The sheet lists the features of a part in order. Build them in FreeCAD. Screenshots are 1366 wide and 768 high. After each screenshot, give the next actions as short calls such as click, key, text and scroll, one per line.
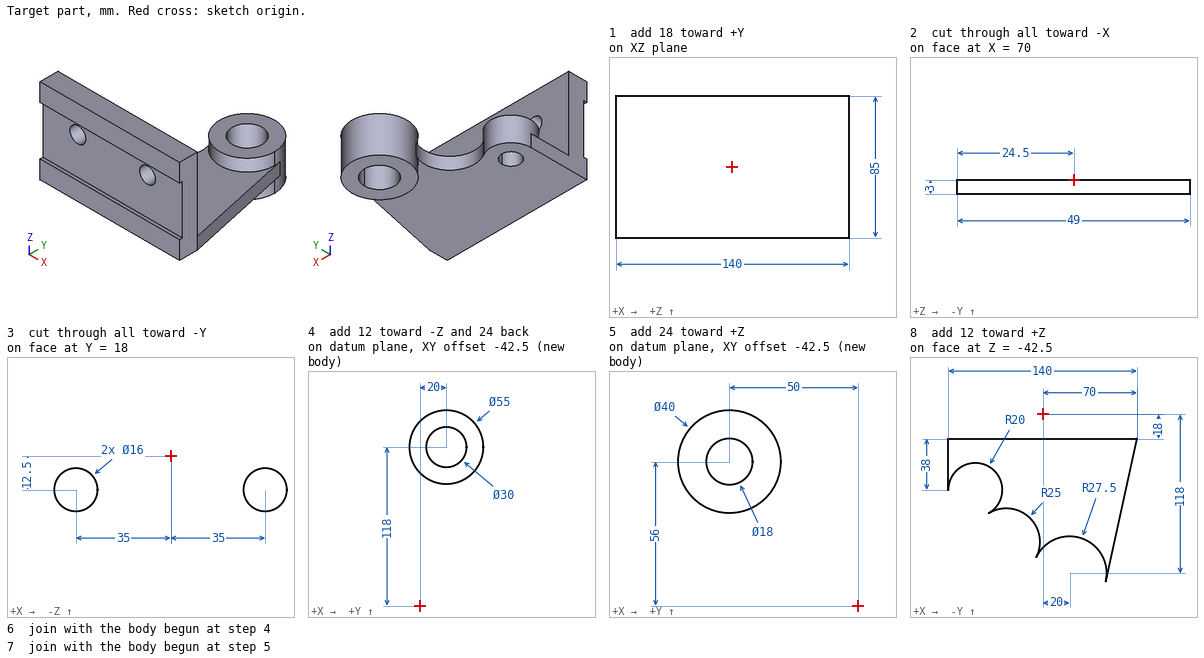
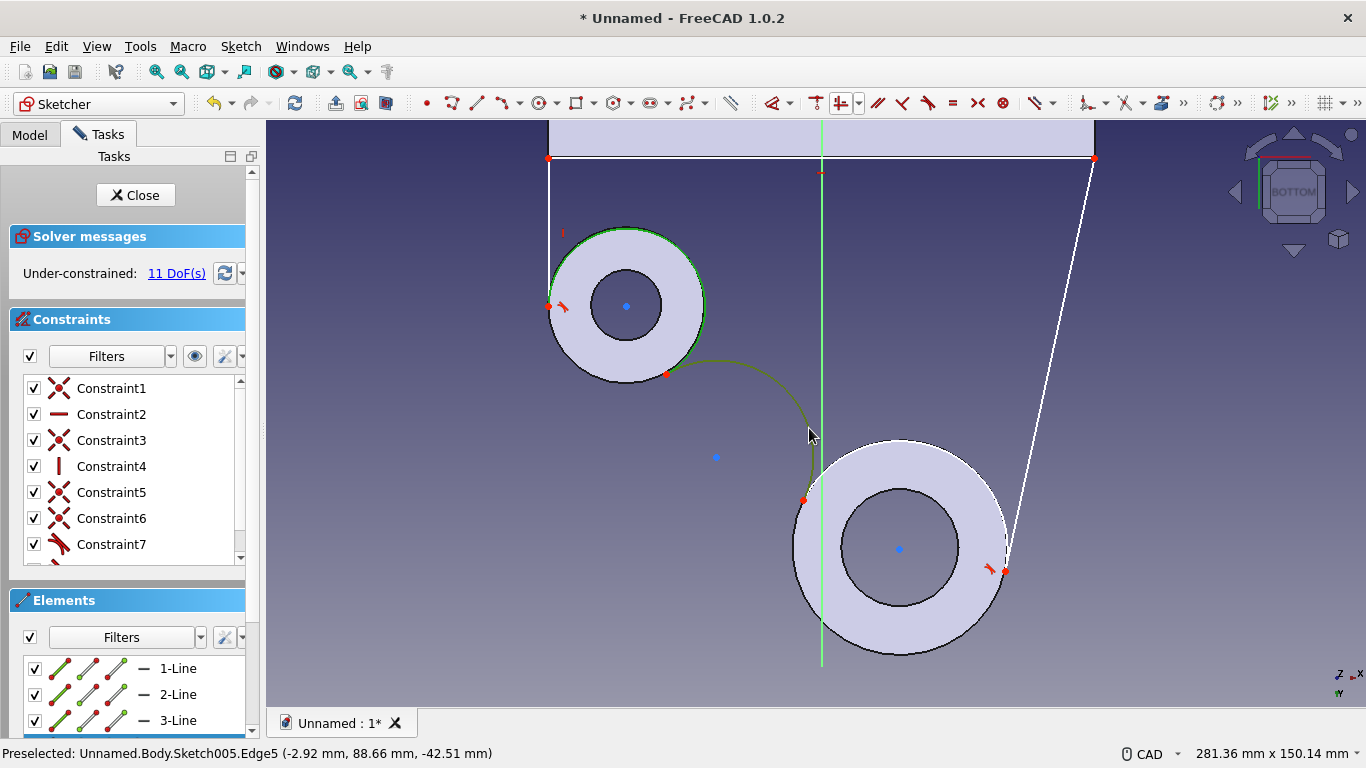
click(928, 104)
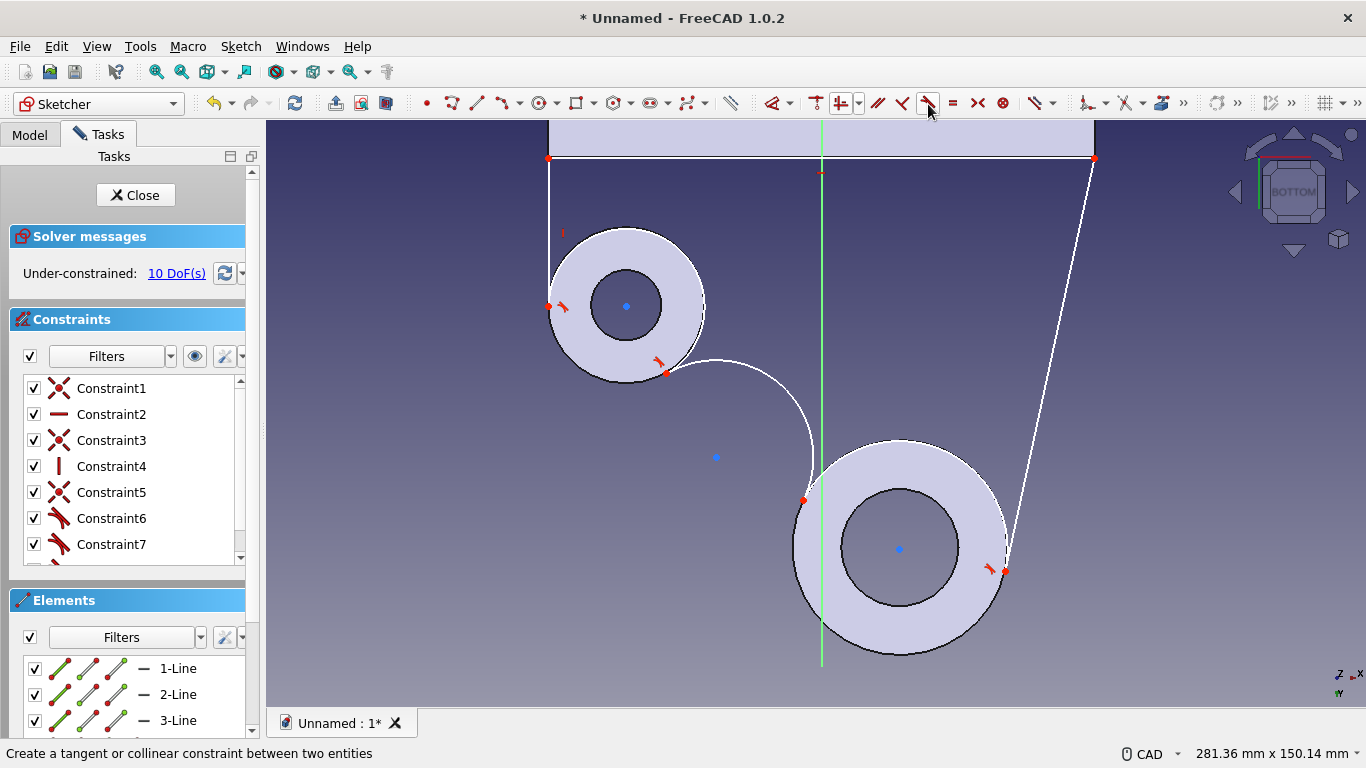
click(809, 428)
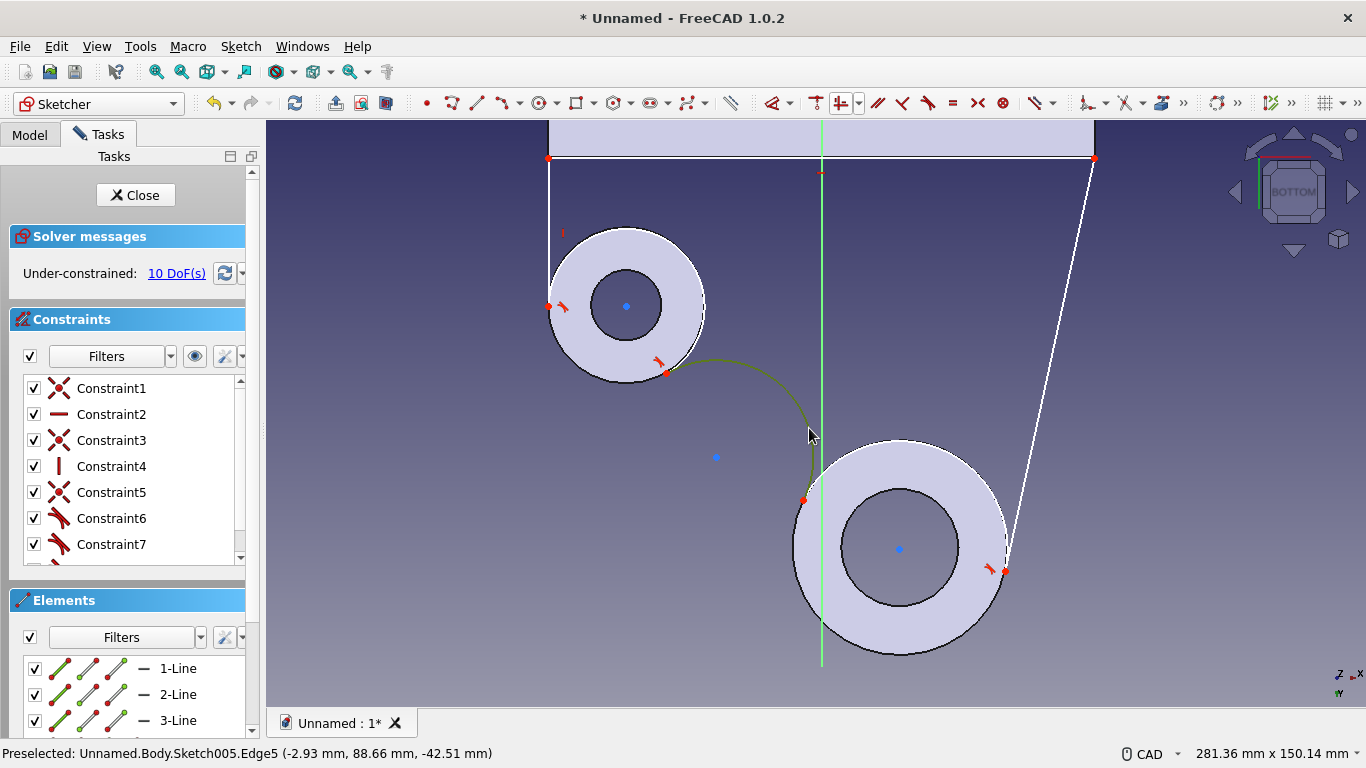
click(985, 483)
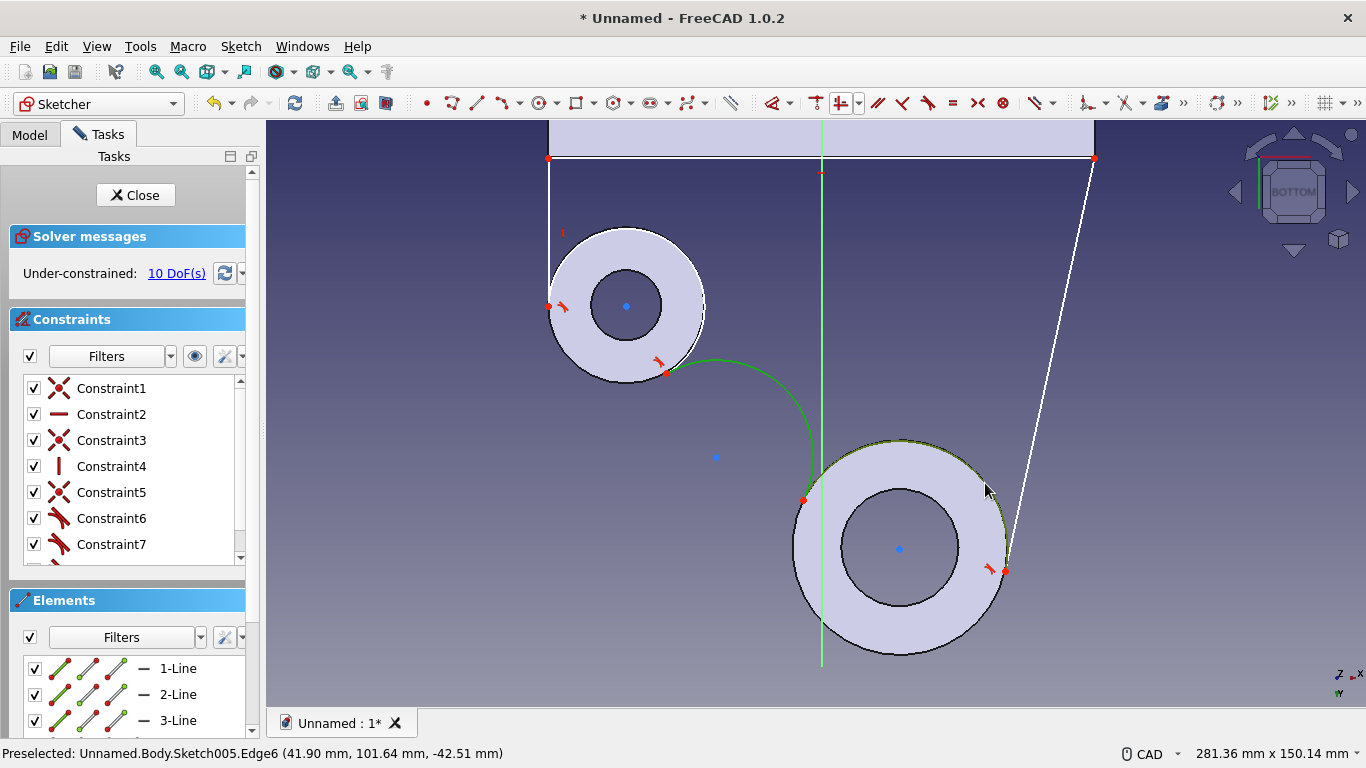
click(928, 104)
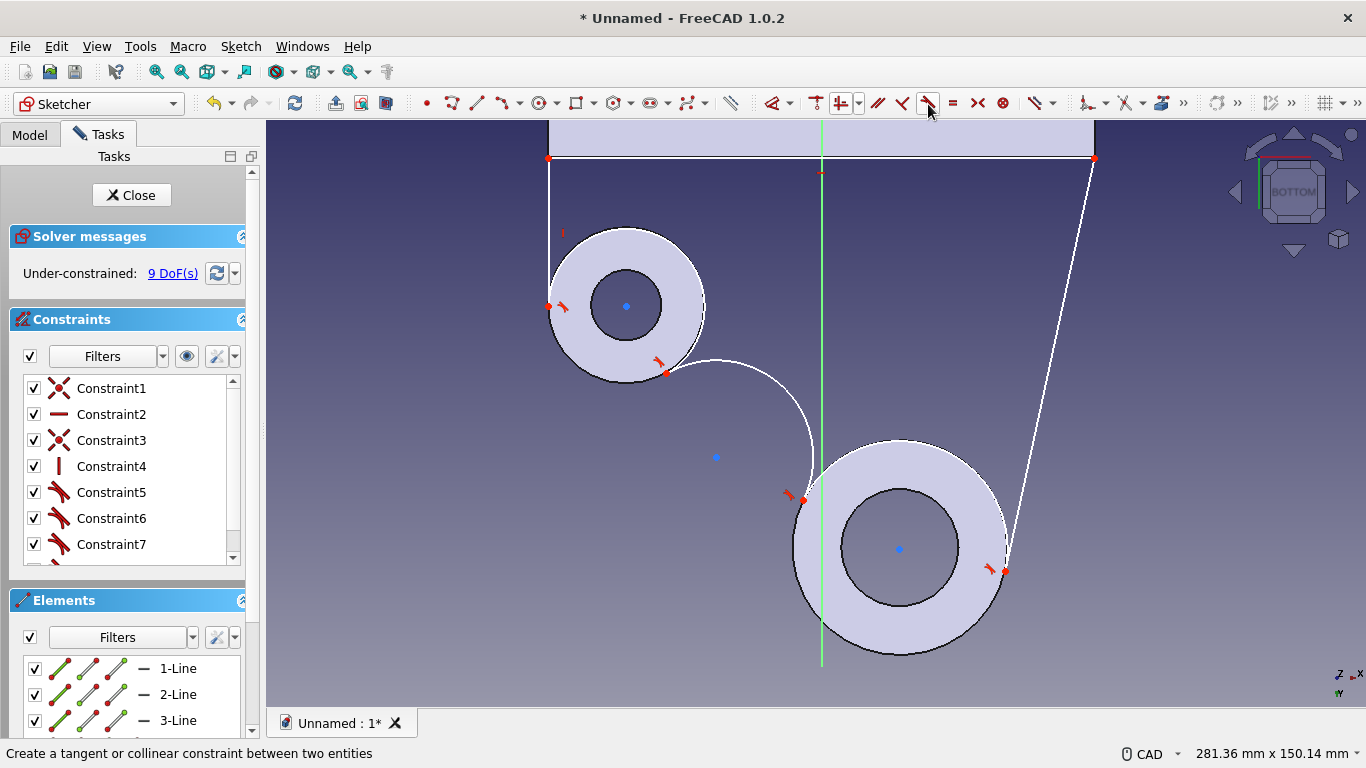
click(772, 104)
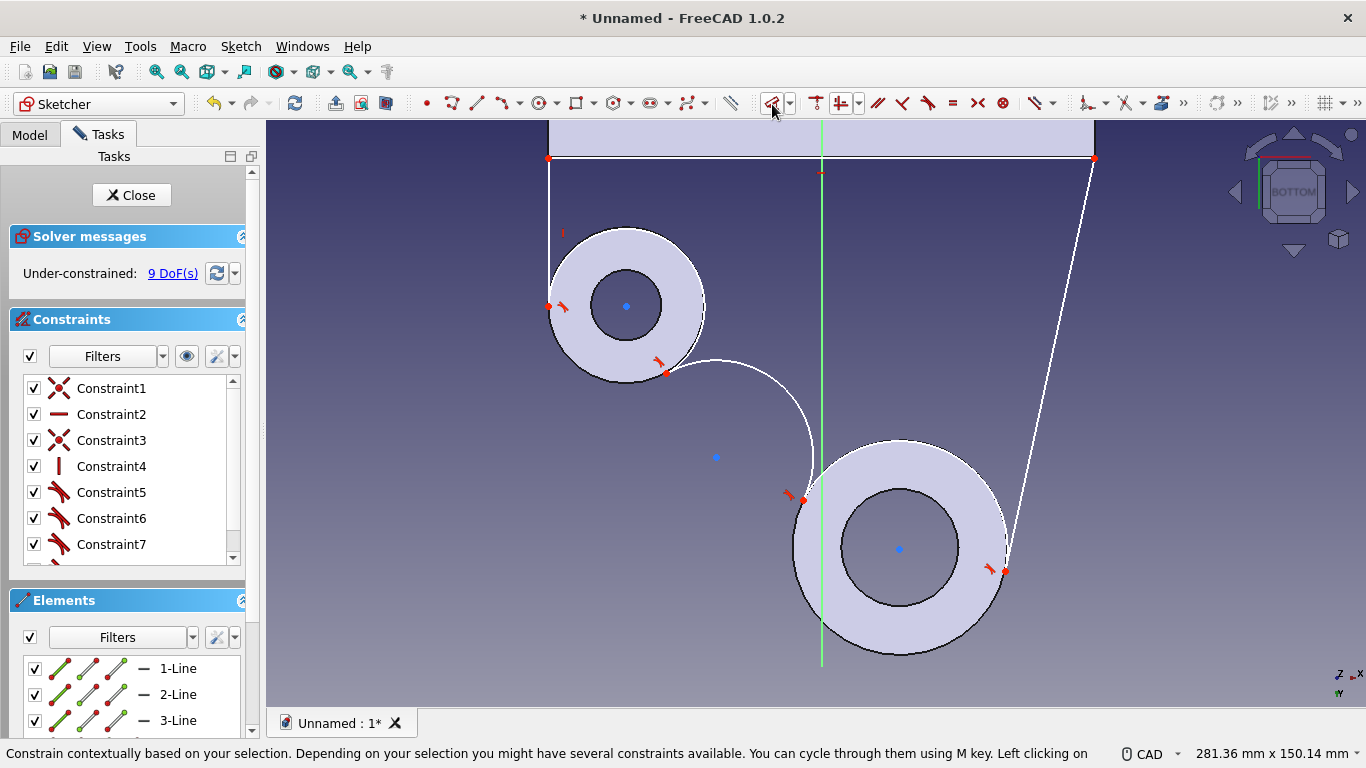
click(703, 290)
click(734, 283)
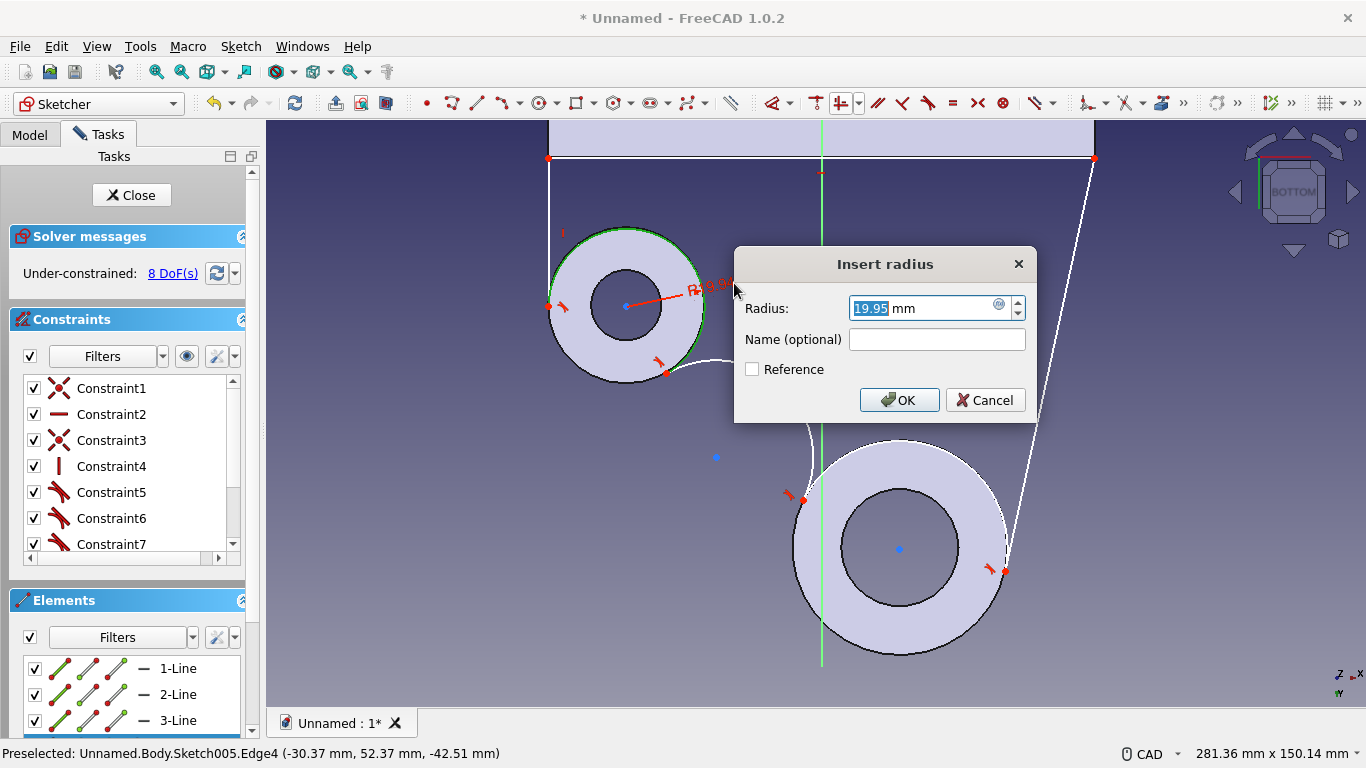
text(20)
key(Return)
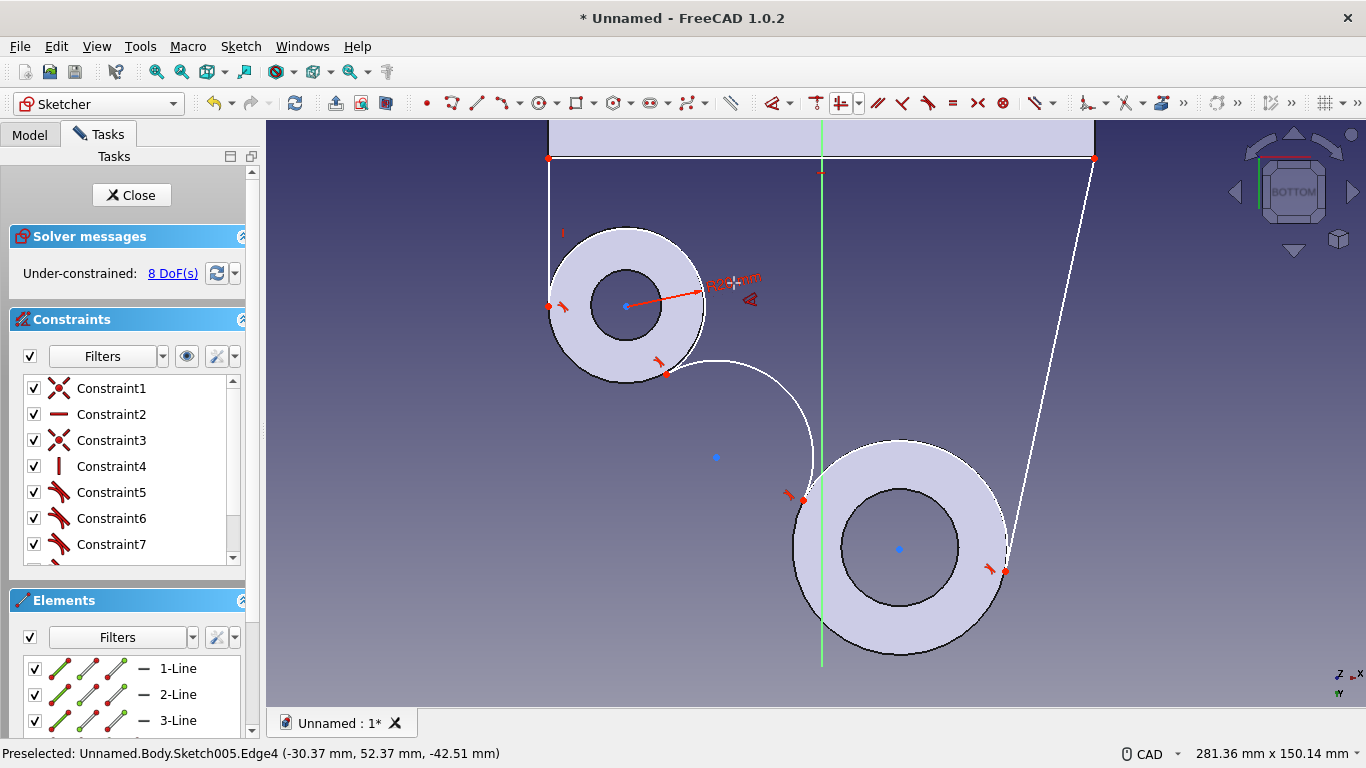
click(809, 428)
click(840, 418)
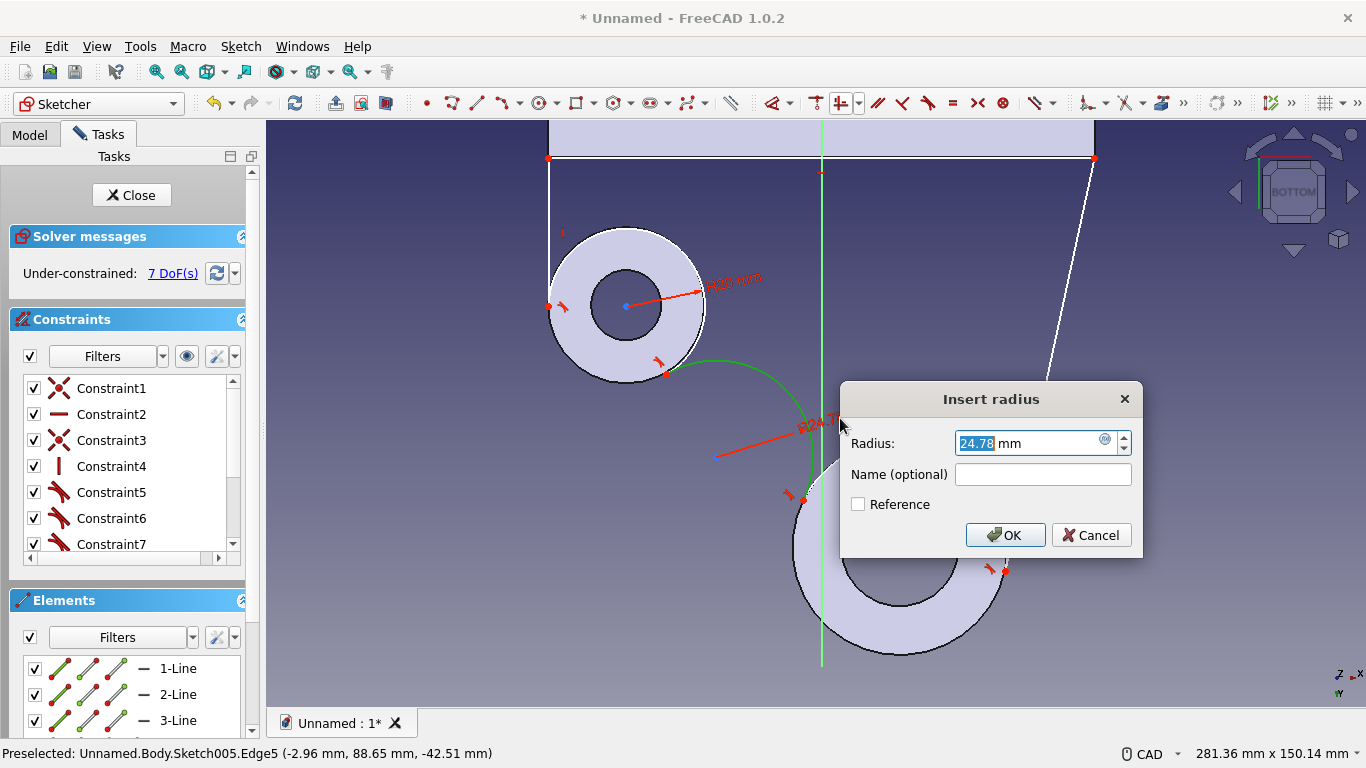
text(25)
key(Return)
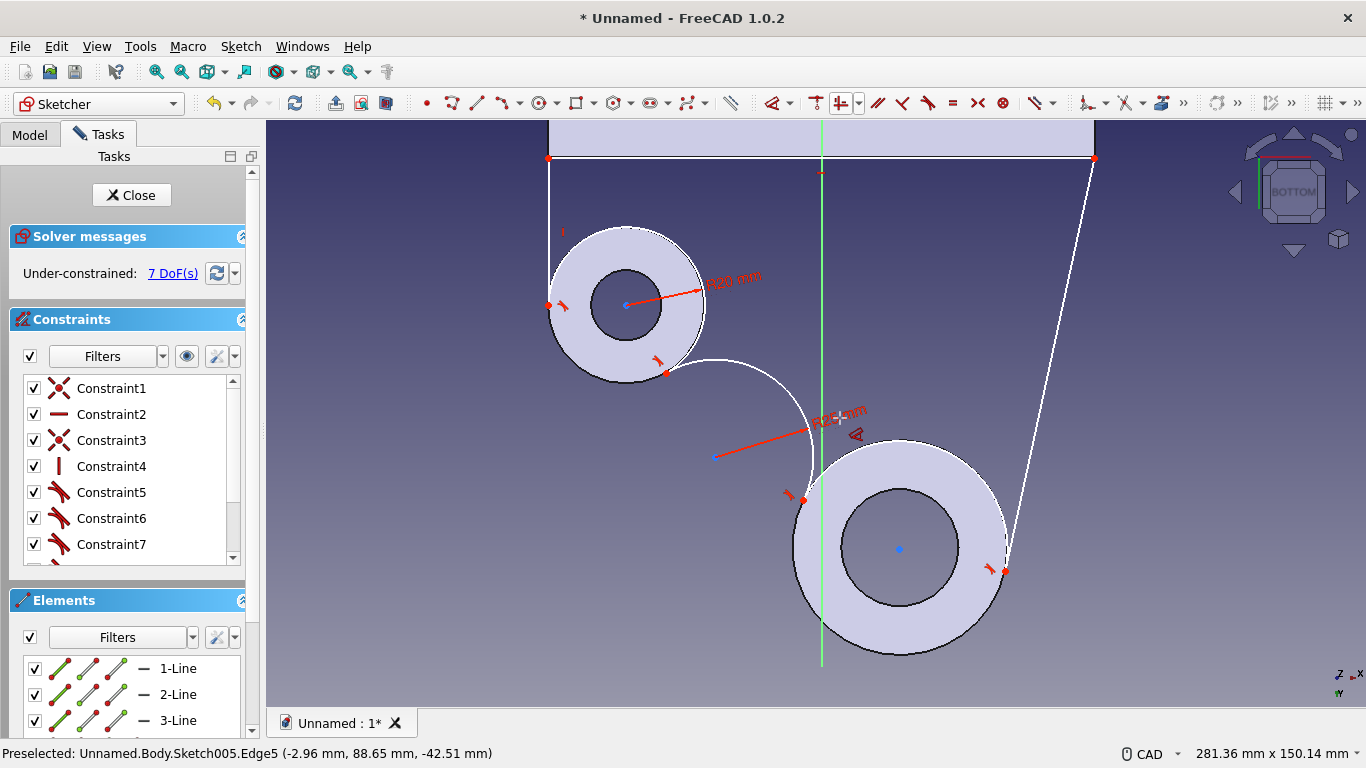
click(985, 483)
click(1010, 463)